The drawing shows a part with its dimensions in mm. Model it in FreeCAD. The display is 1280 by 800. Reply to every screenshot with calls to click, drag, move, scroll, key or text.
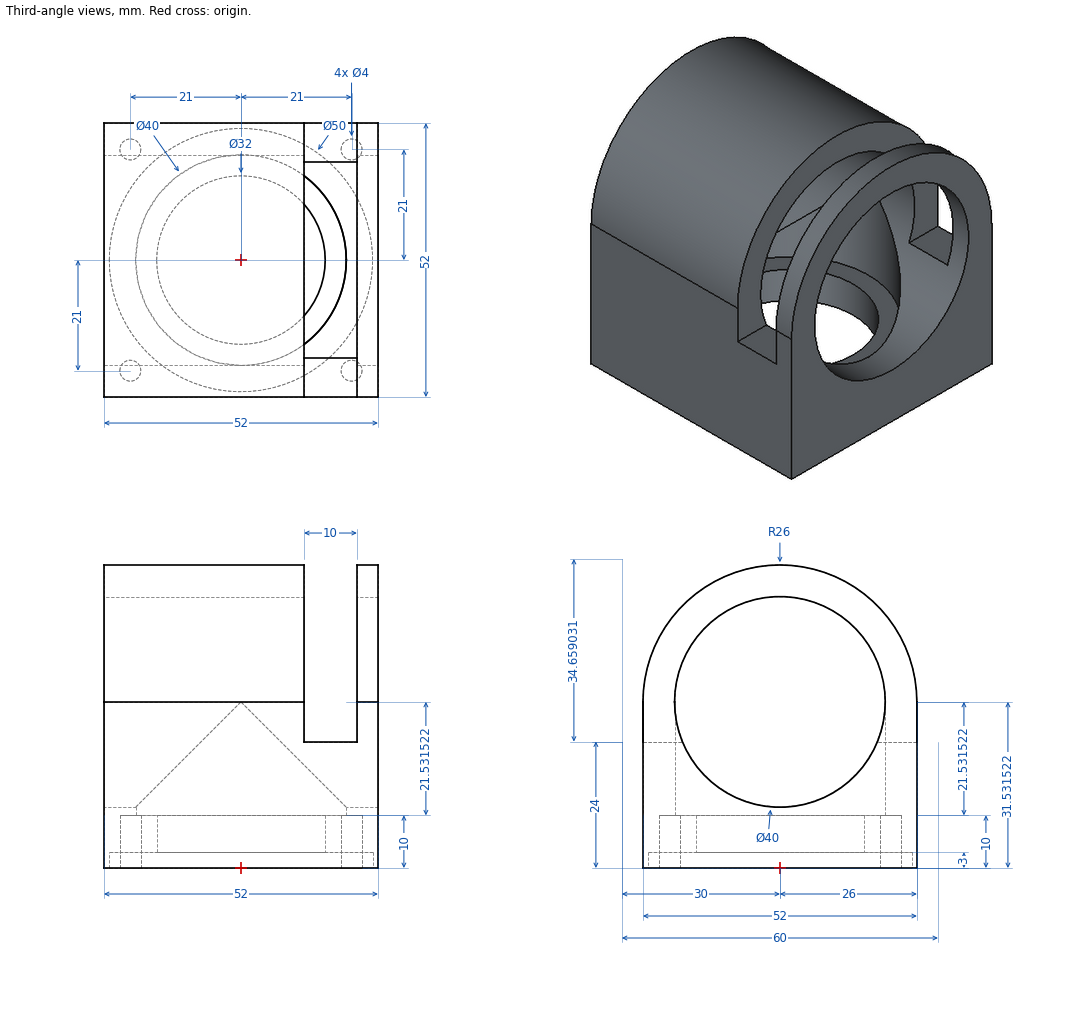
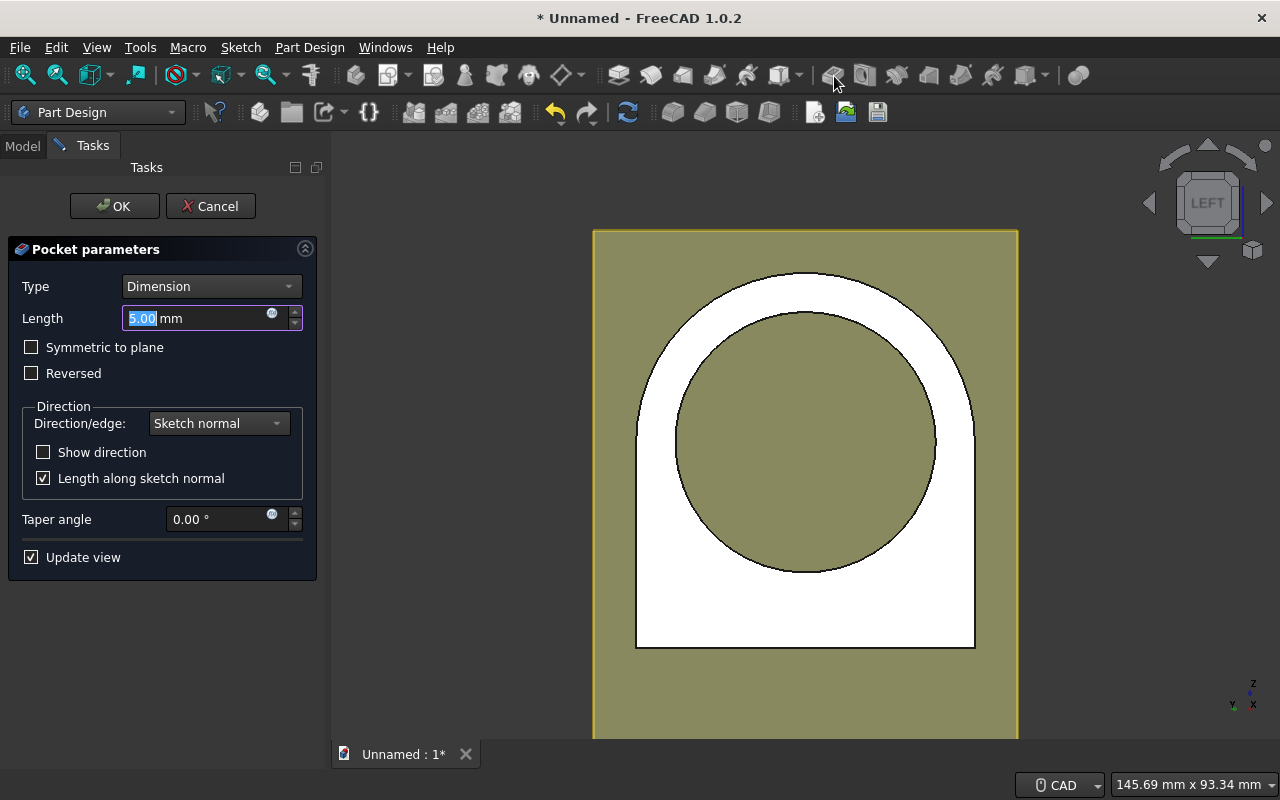
text(10)
key(Tab)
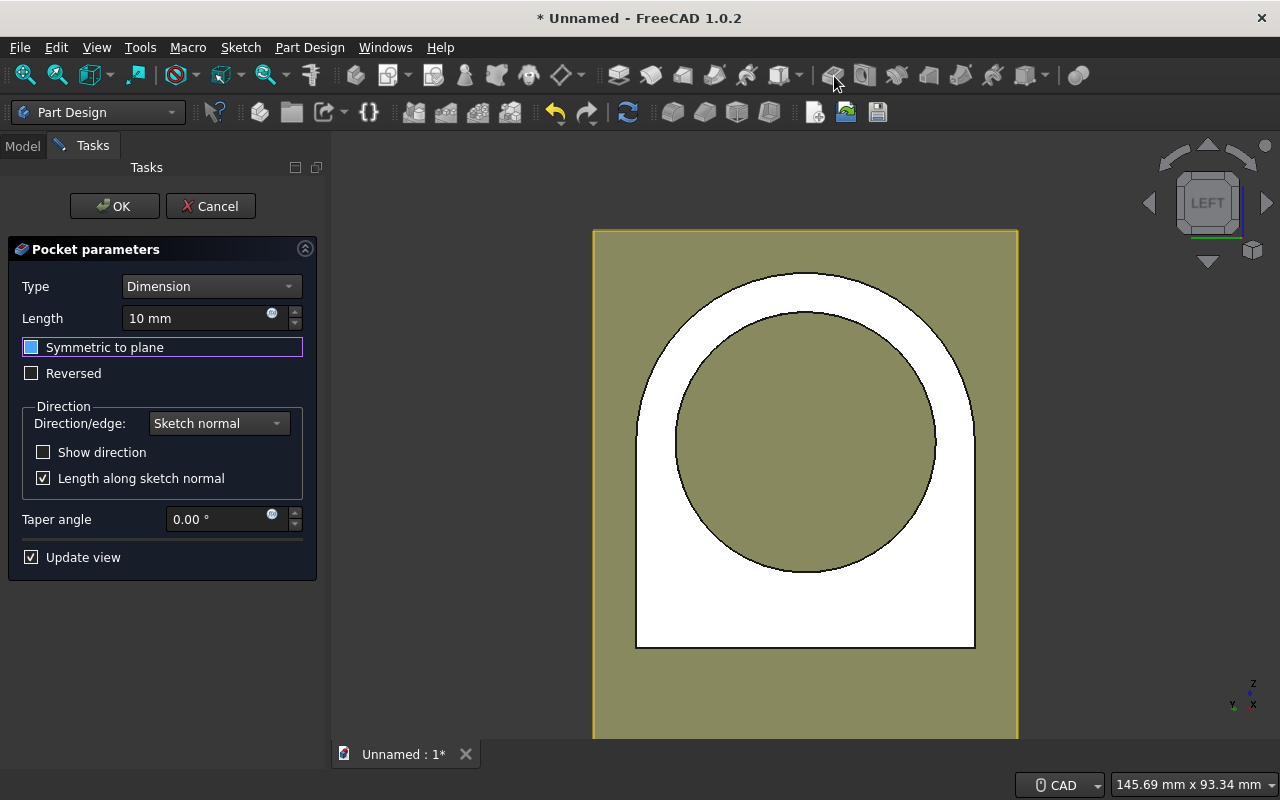
click(115, 206)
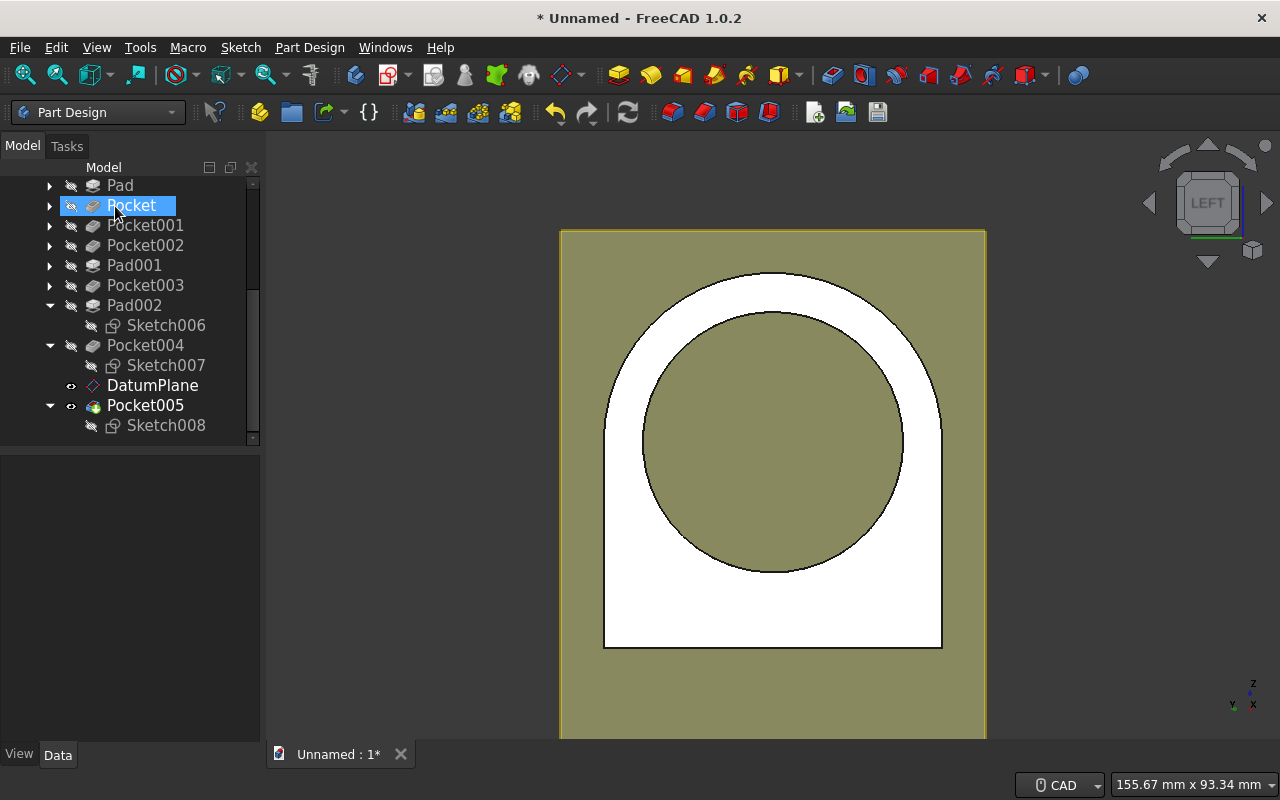
click(116, 386)
key(space)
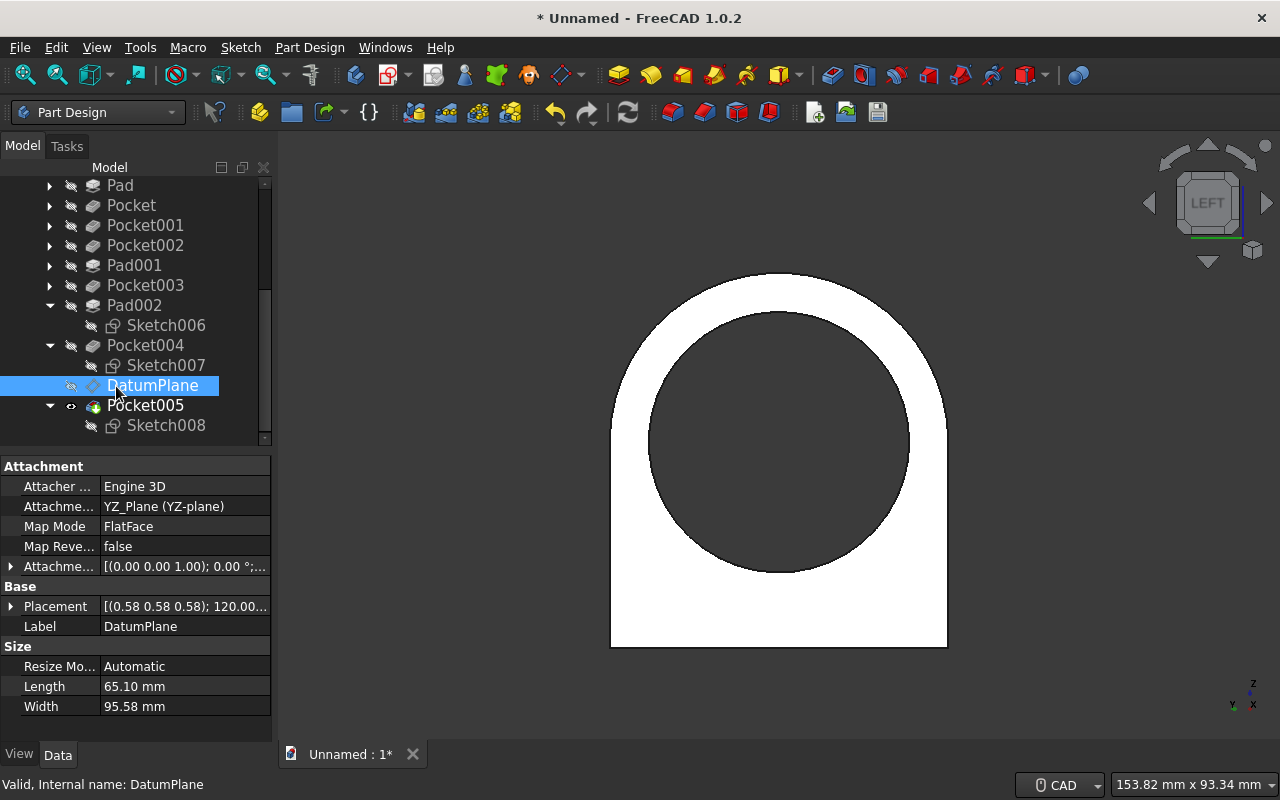
key(0)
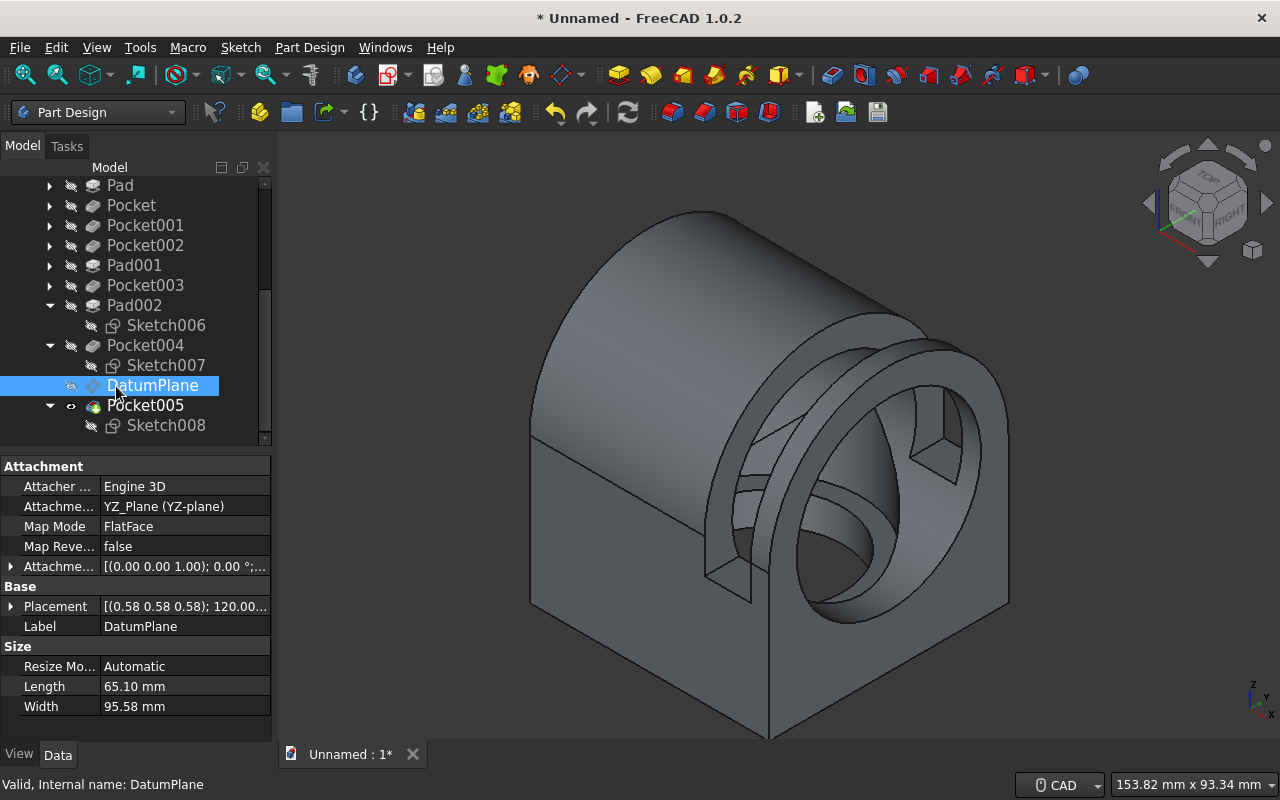
click(26, 76)